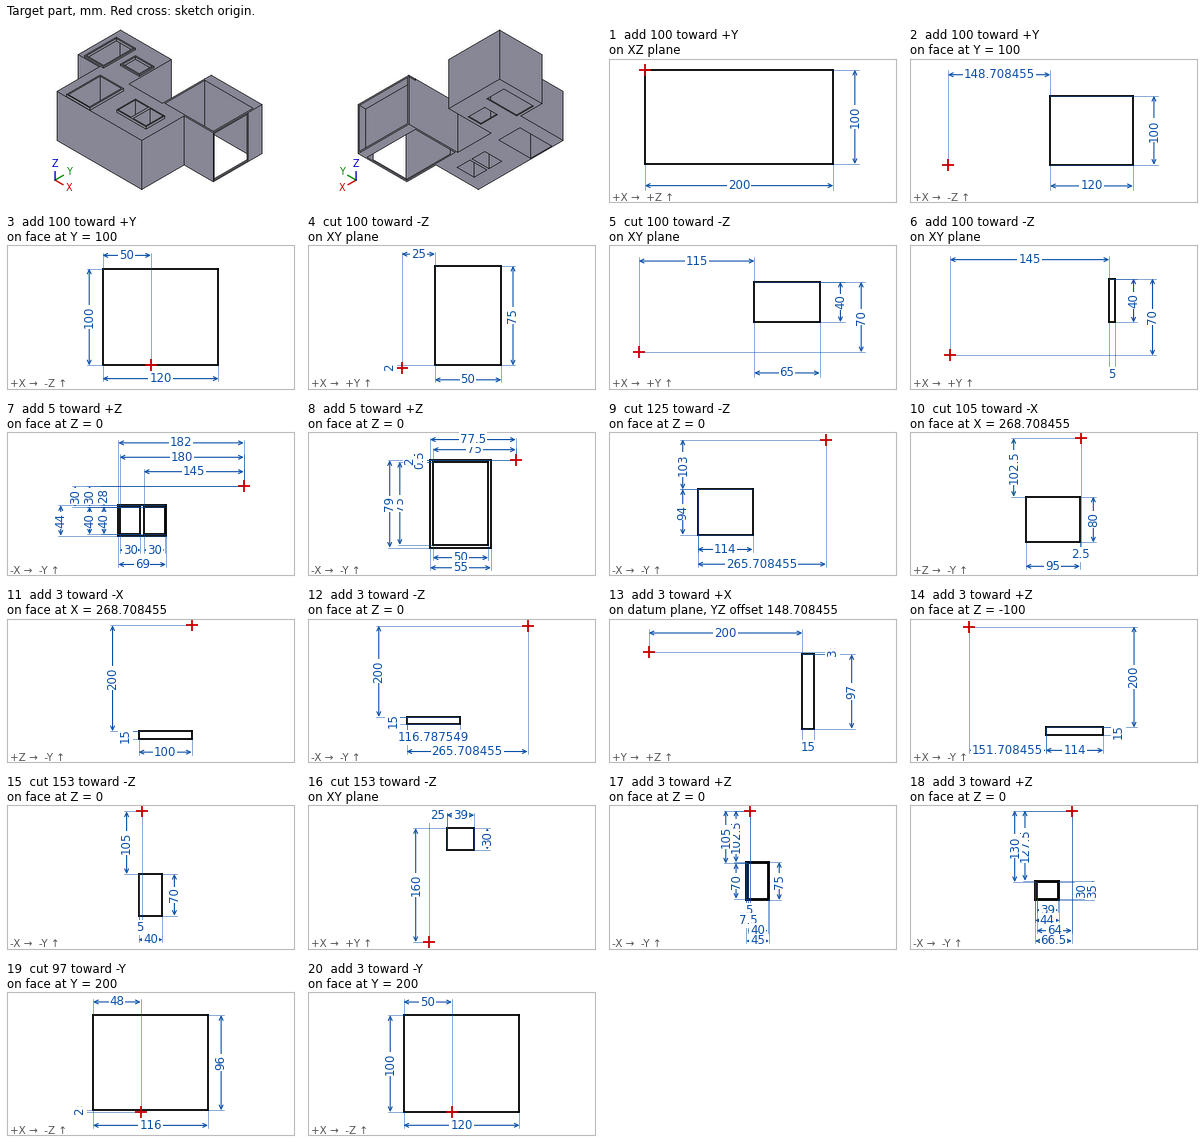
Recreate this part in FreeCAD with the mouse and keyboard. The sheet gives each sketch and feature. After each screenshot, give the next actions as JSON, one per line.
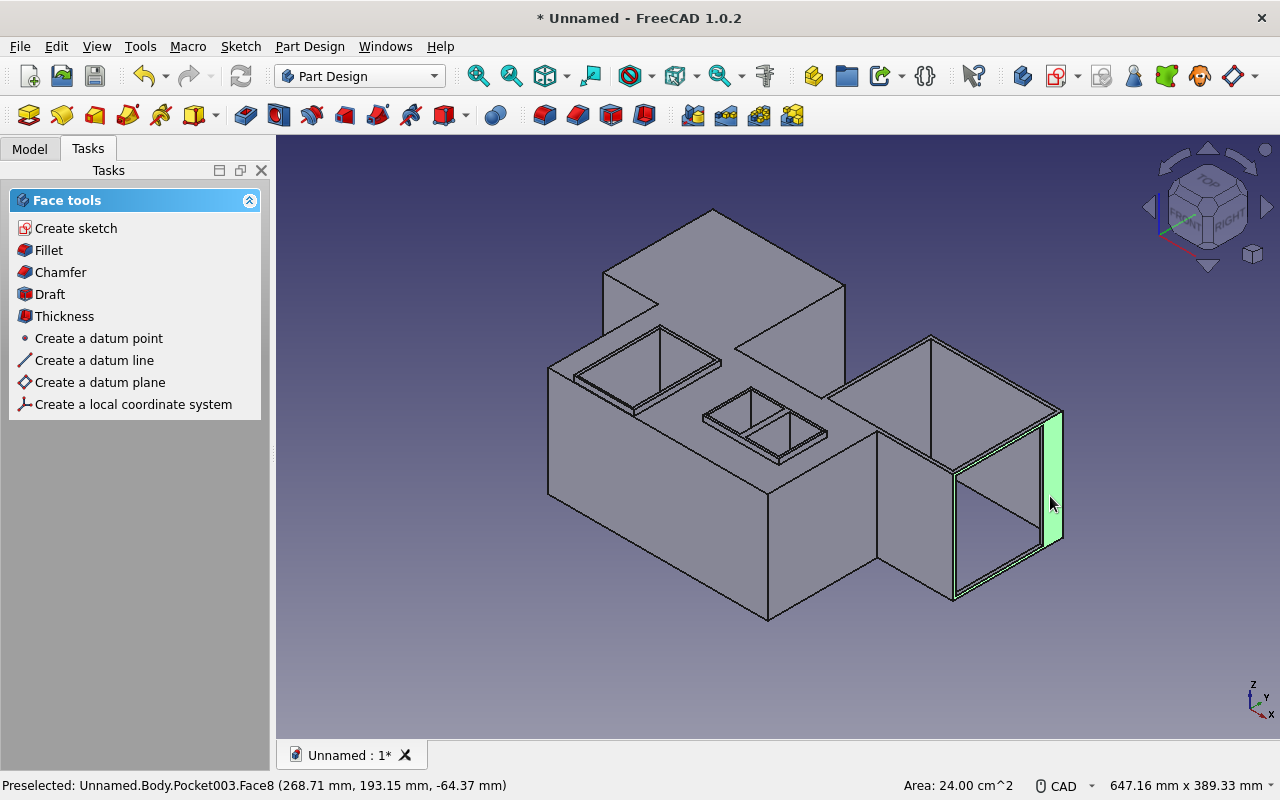
{"action": "left_click", "coordinate": [1056, 76]}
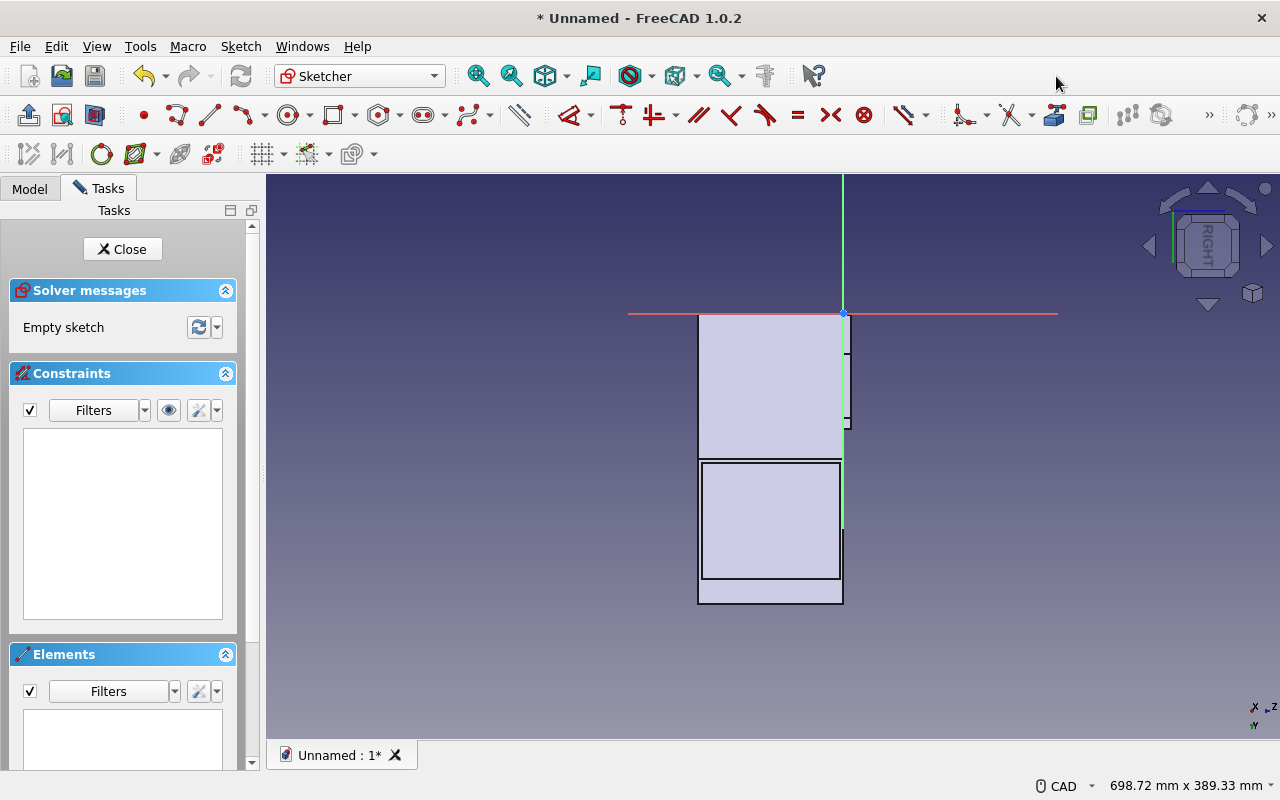
{"action": "left_click", "coordinate": [332, 116]}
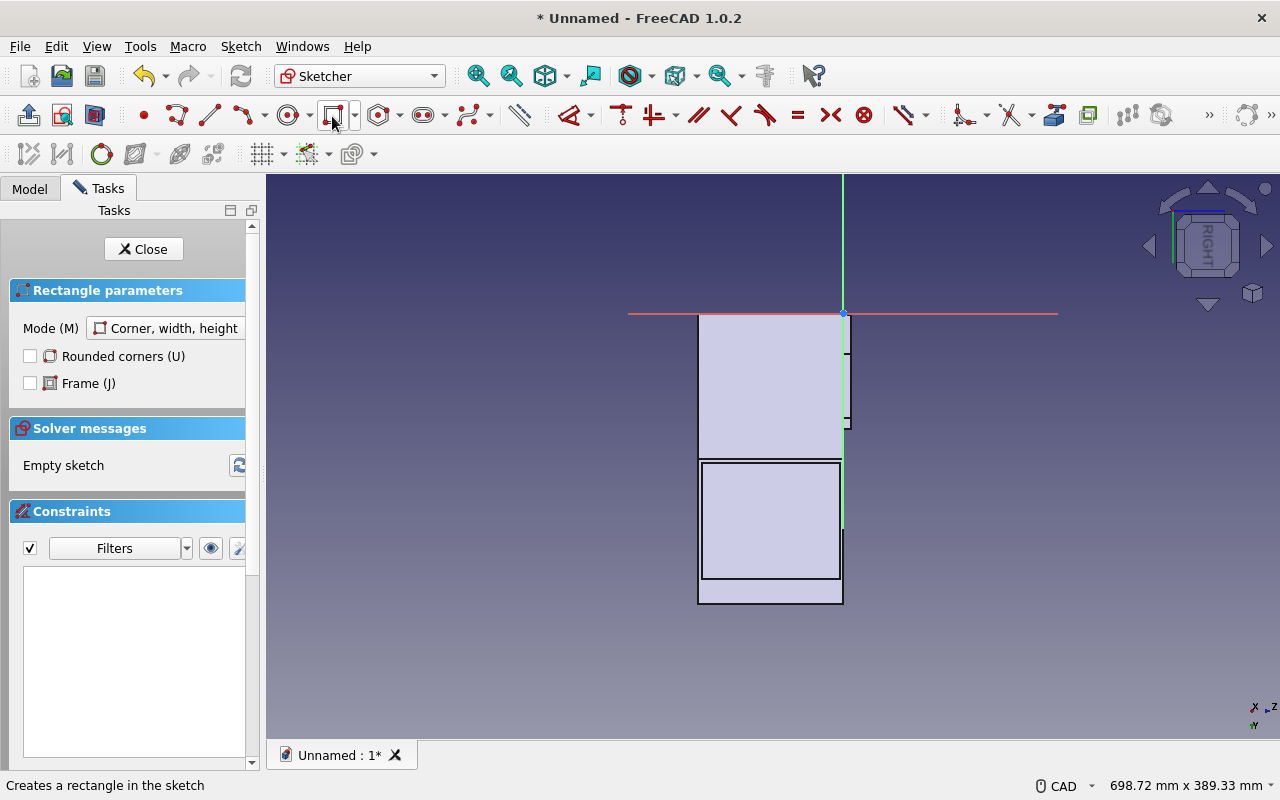
{"action": "left_click", "coordinate": [698, 604]}
{"action": "left_click", "coordinate": [843, 626]}
{"action": "key", "text": "Escape"}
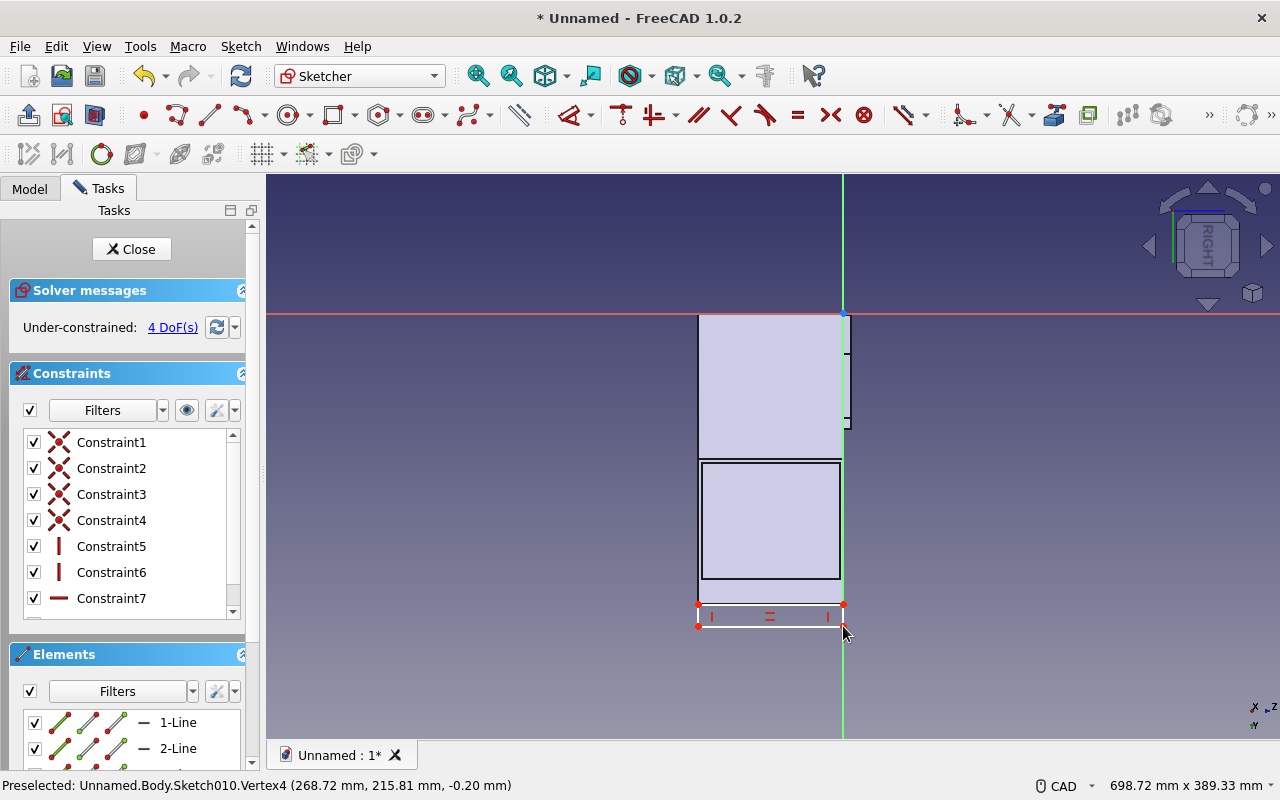
{"action": "left_click", "coordinate": [843, 627]}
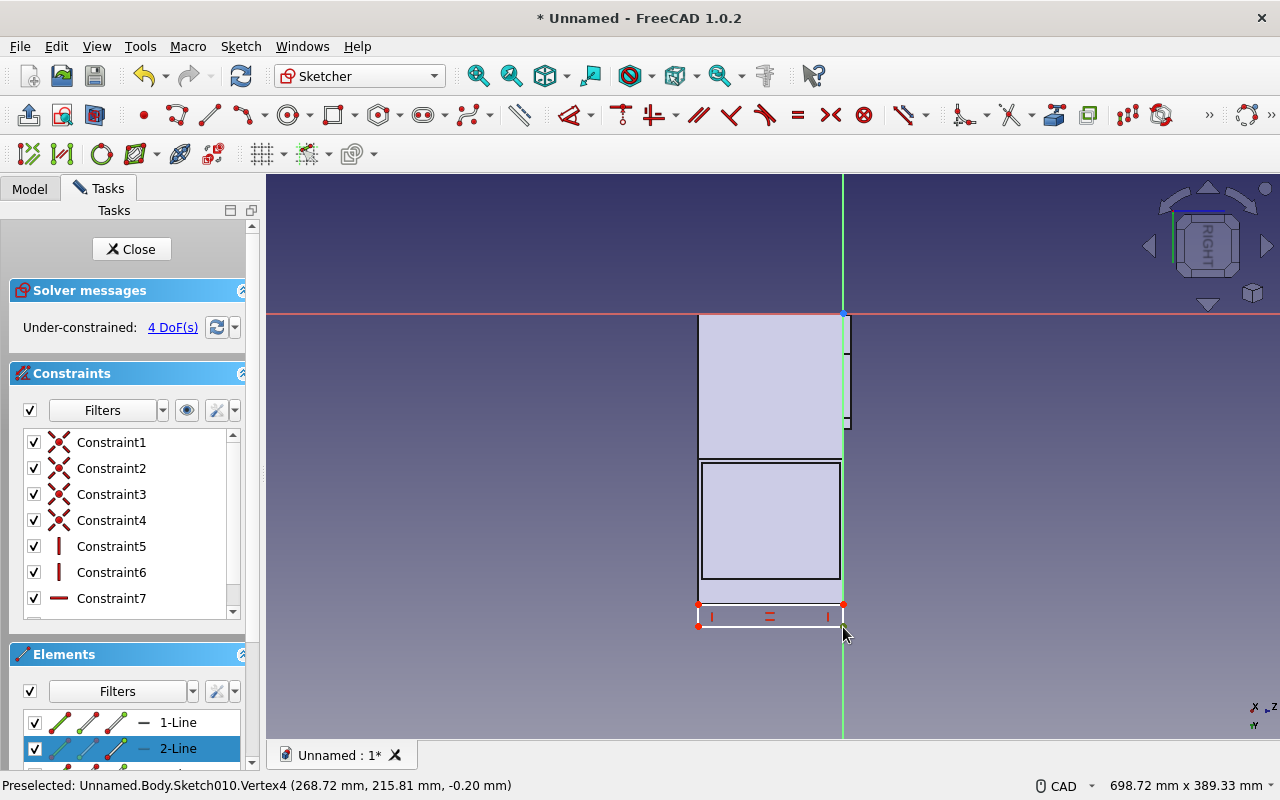
{"action": "left_click", "coordinate": [843, 675]}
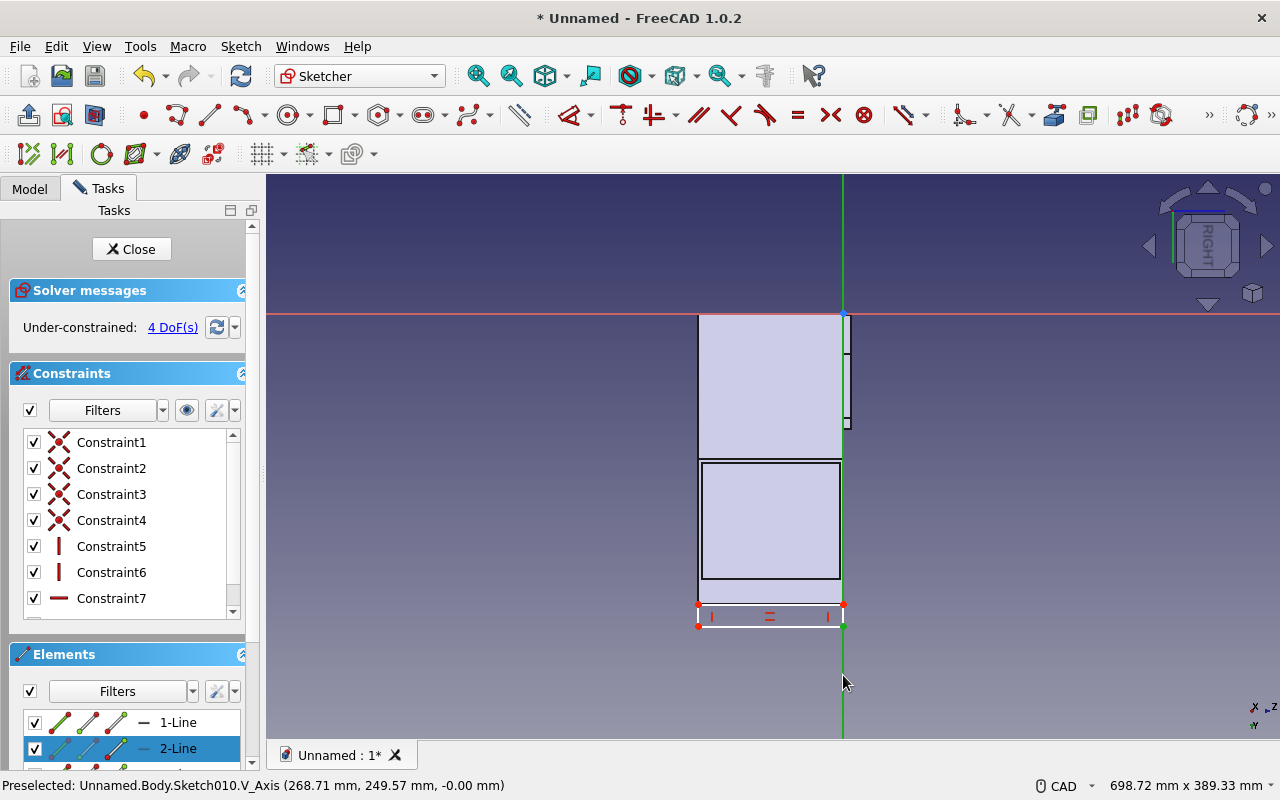
{"action": "left_click", "coordinate": [621, 116]}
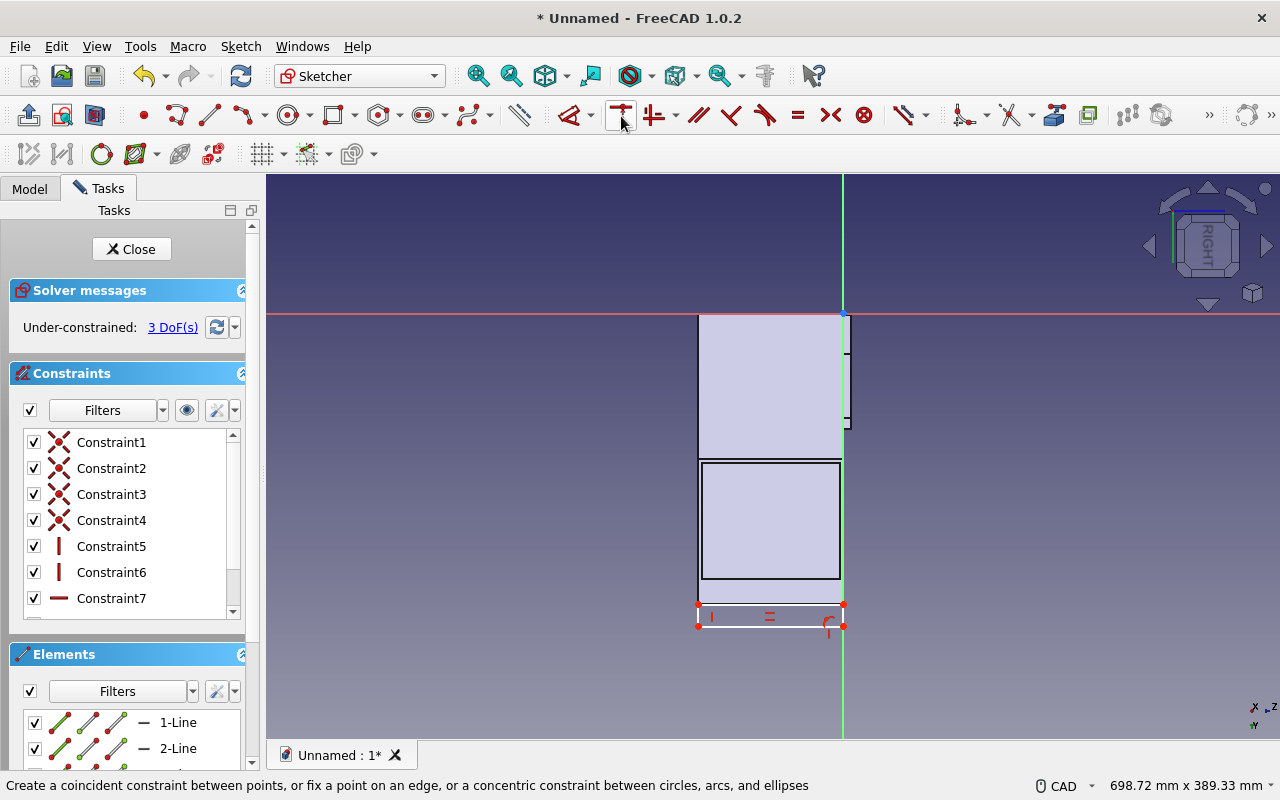
{"action": "left_click", "coordinate": [568, 116]}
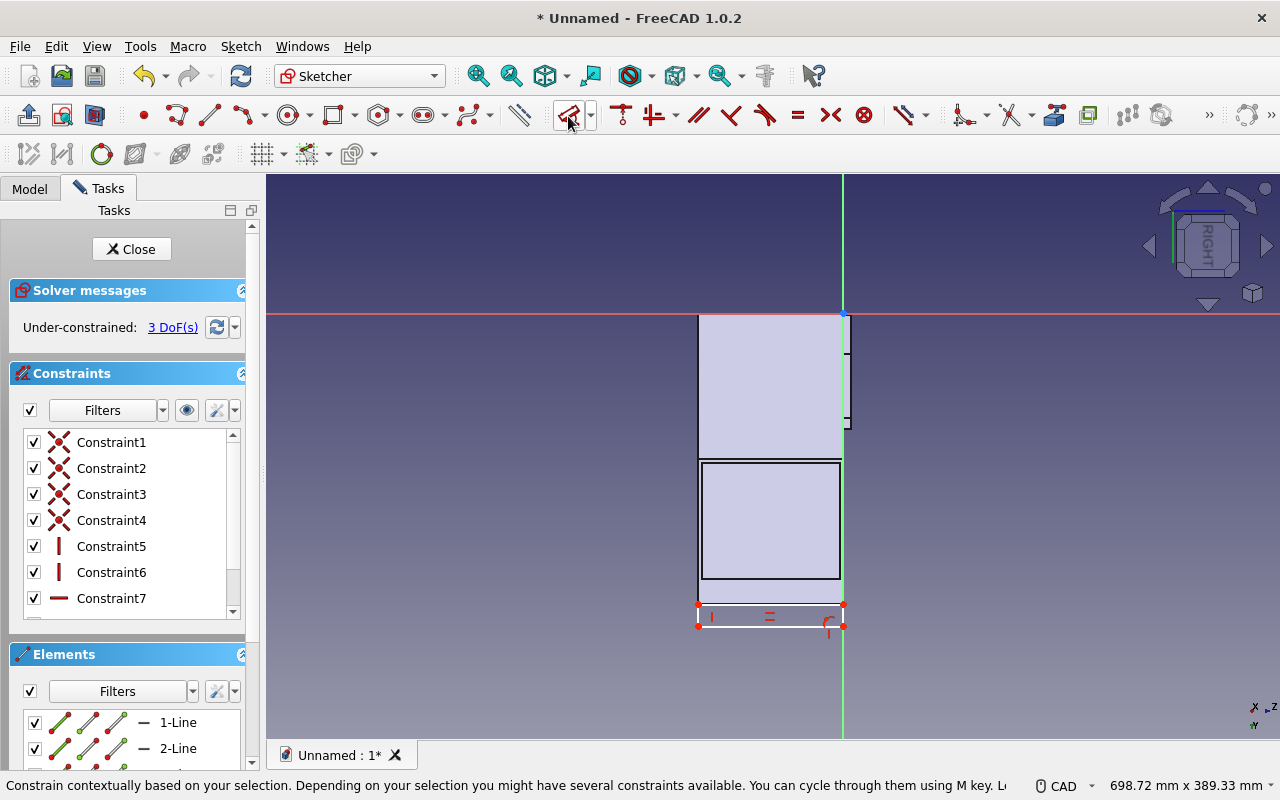
{"action": "scroll", "coordinate": [698, 616], "scroll_direction": "up", "scroll_amount": 4}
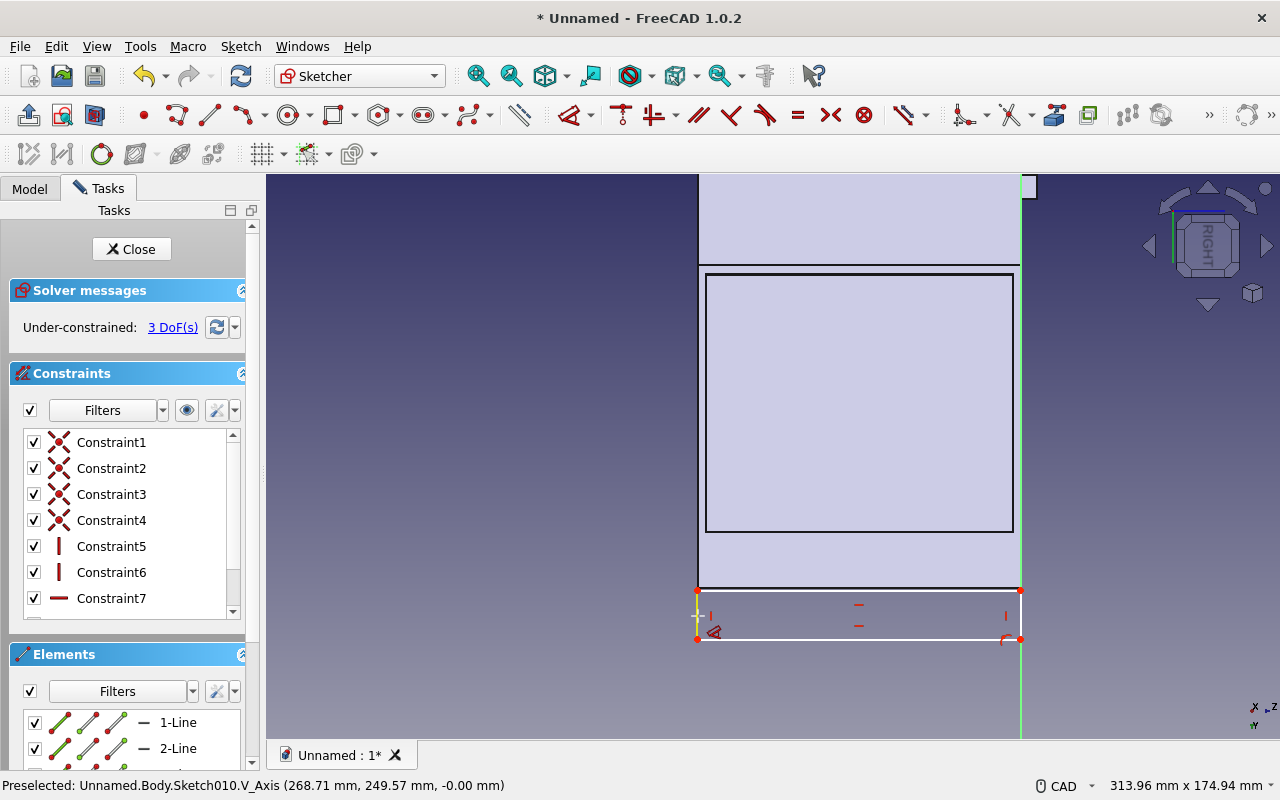
{"action": "left_click", "coordinate": [697, 615]}
{"action": "left_click", "coordinate": [663, 615]}